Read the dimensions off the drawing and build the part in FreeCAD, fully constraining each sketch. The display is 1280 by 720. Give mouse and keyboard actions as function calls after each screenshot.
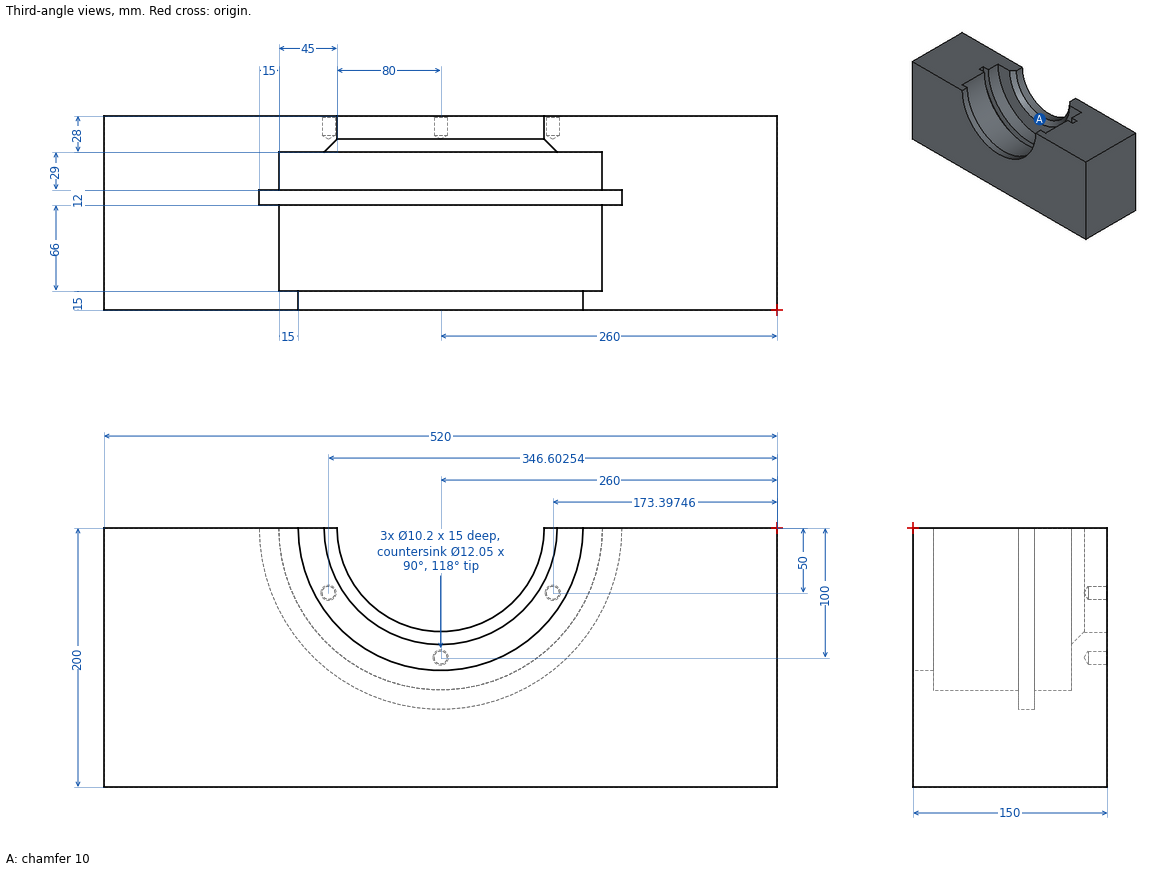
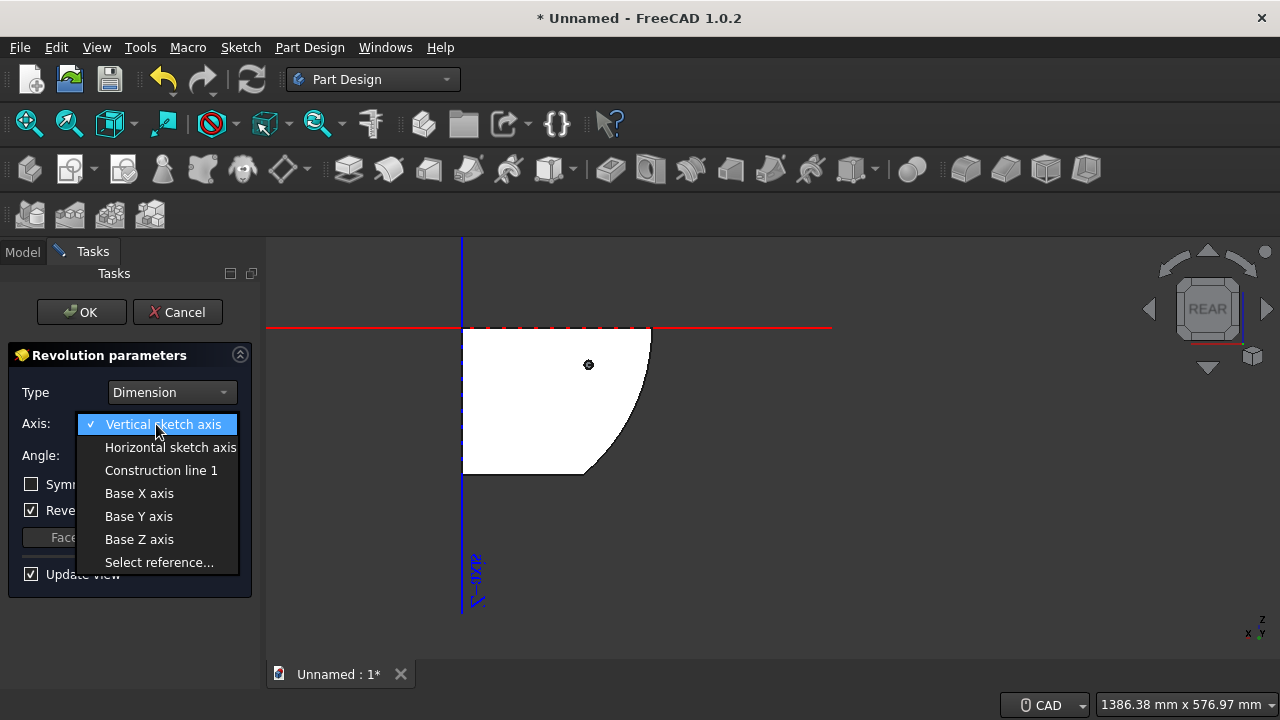
click(156, 470)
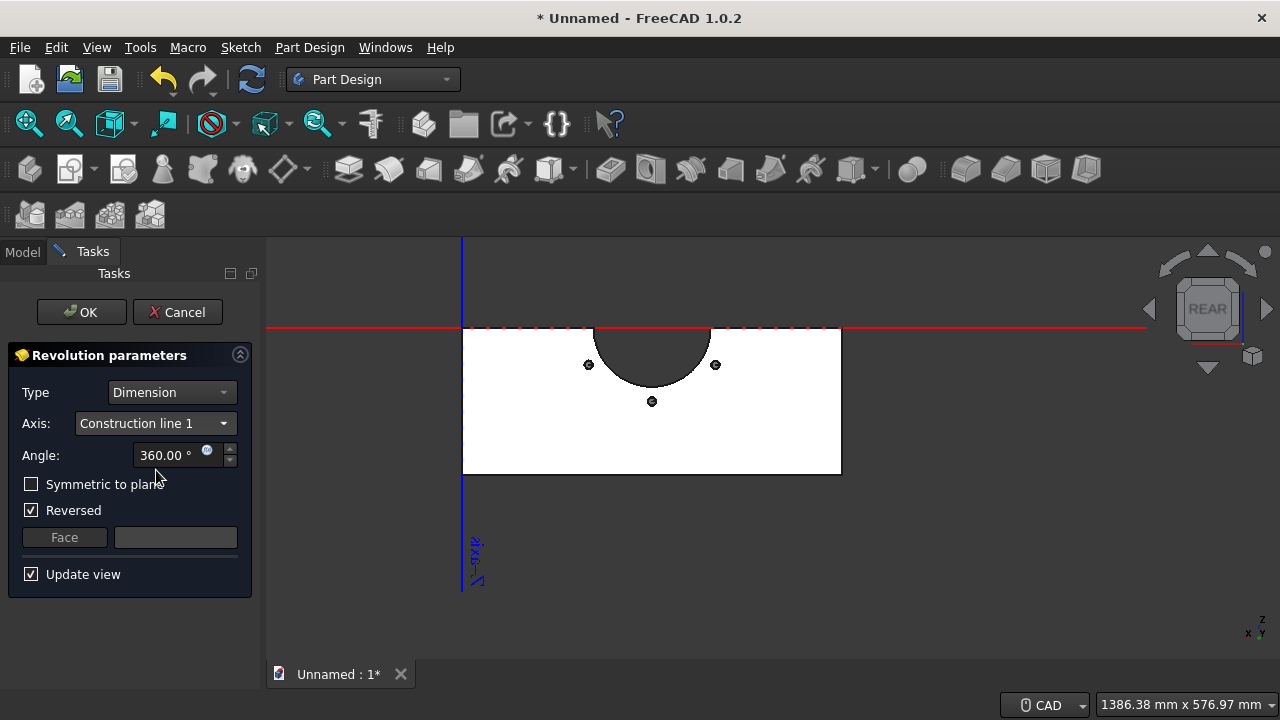
click(82, 312)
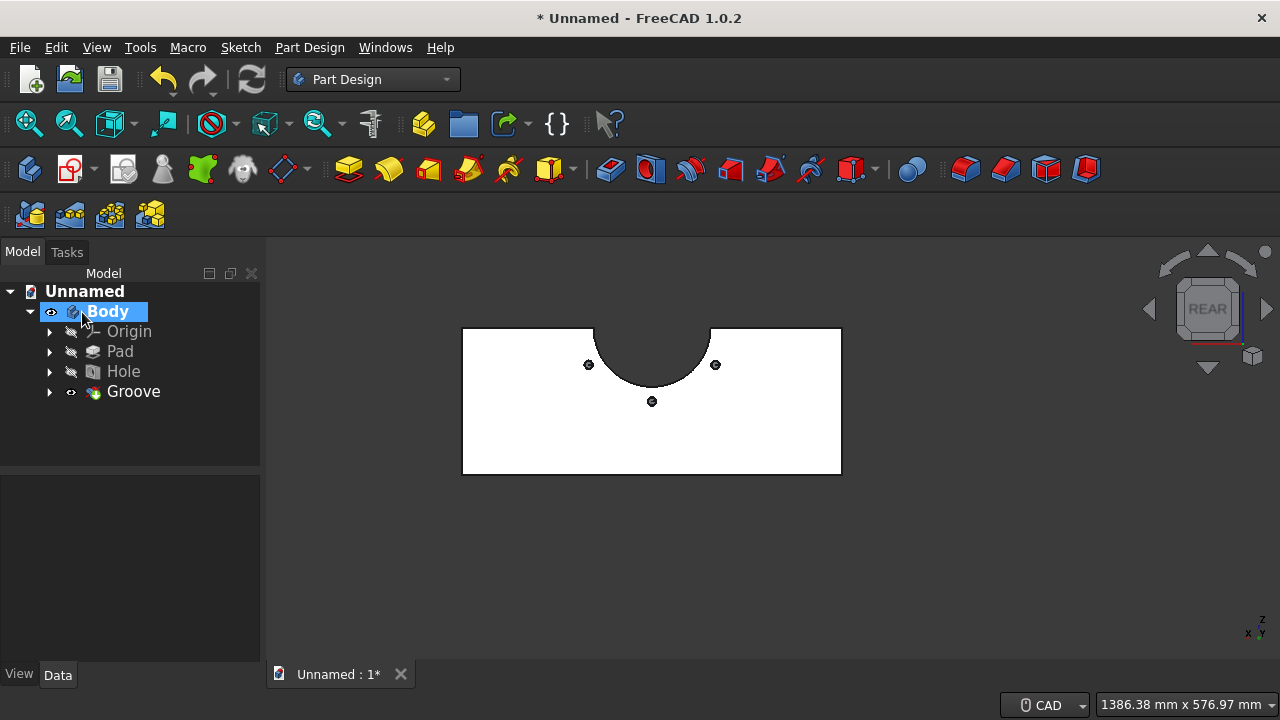
click(30, 124)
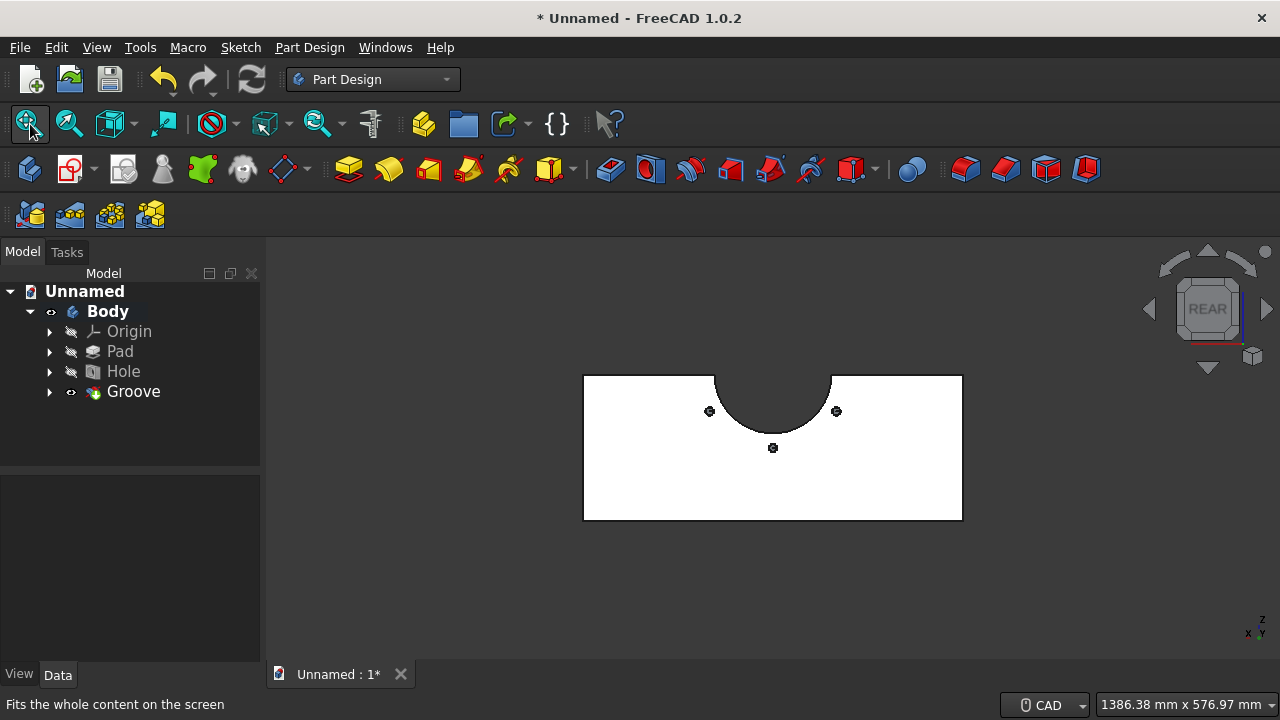
key(0)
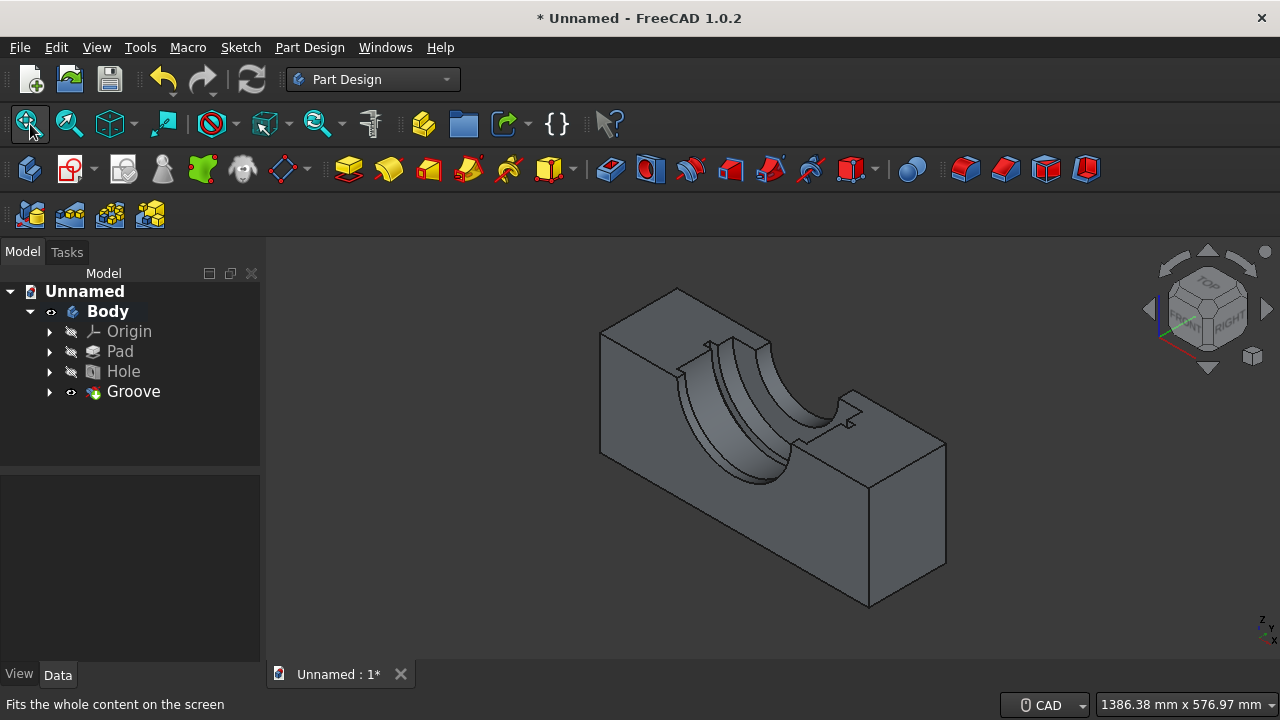
click(797, 421)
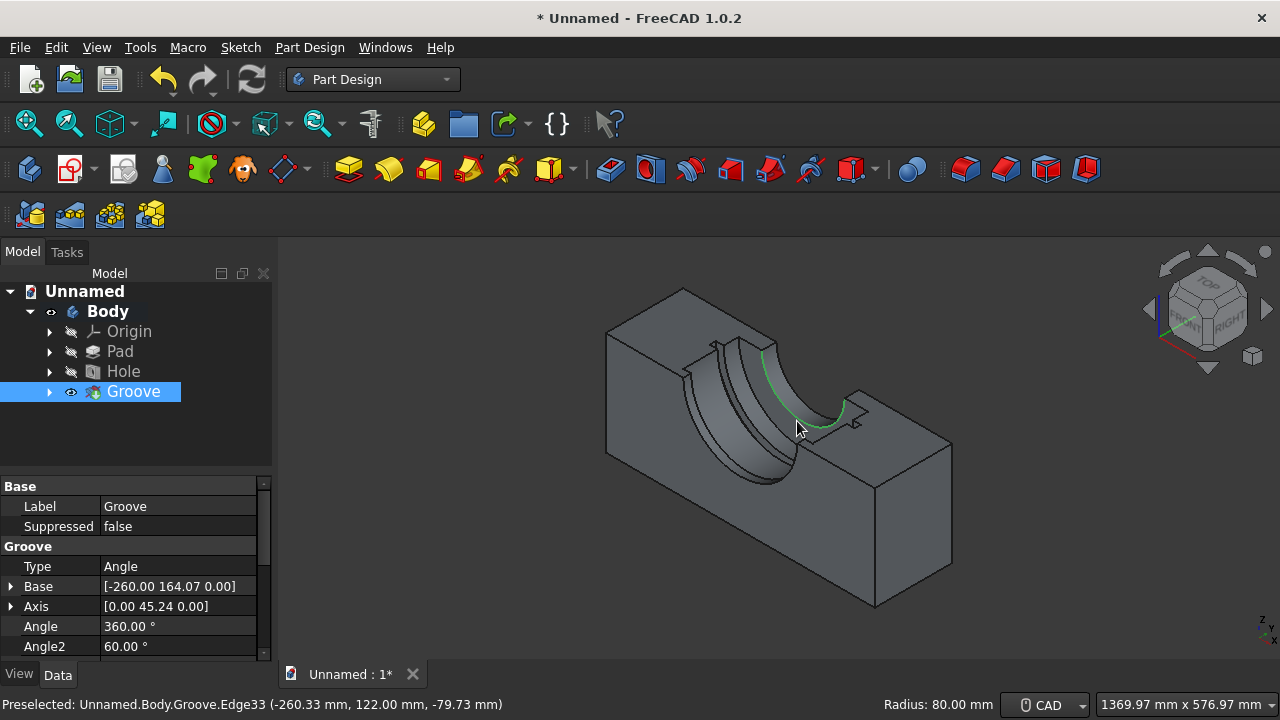
click(1006, 170)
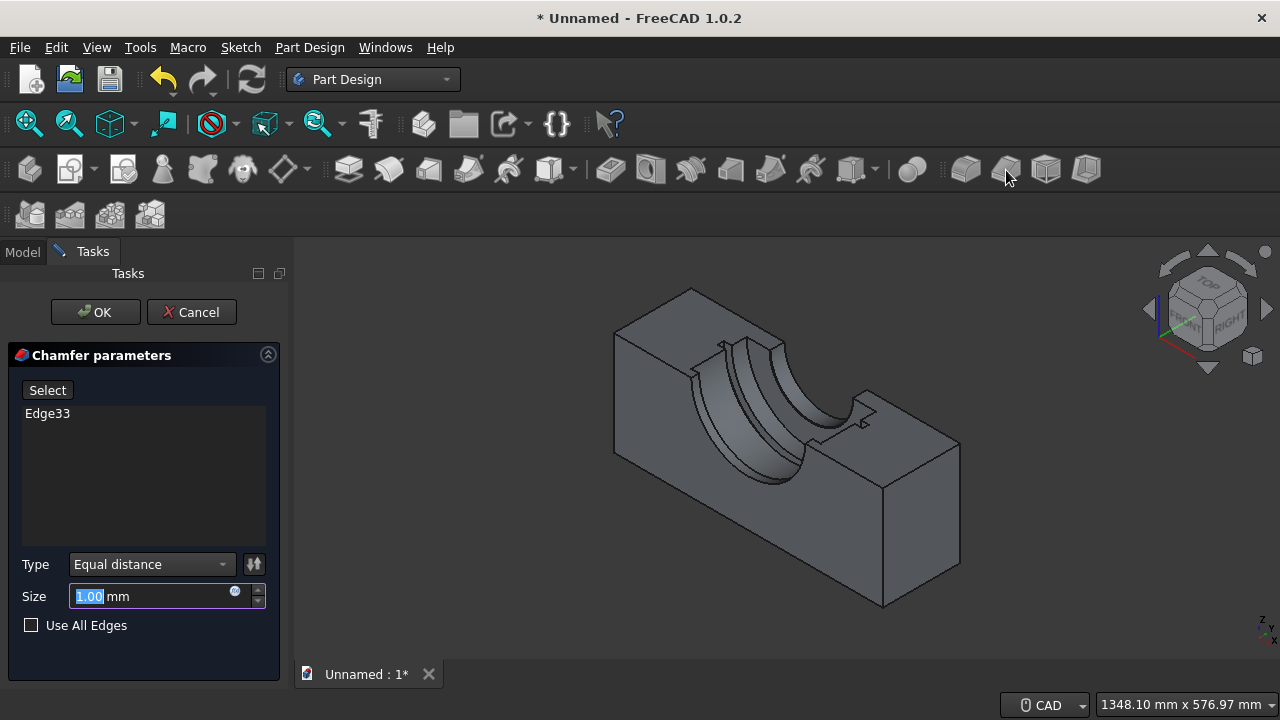
text(10)
key(Tab)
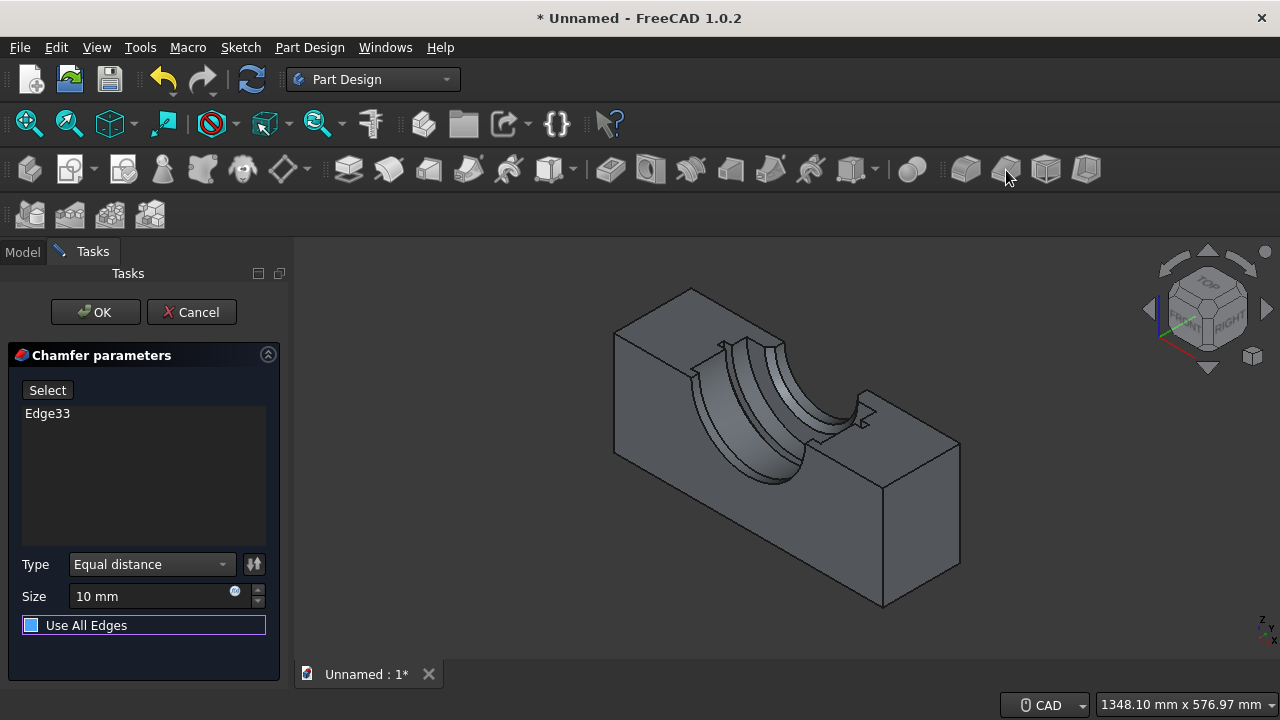
click(96, 312)